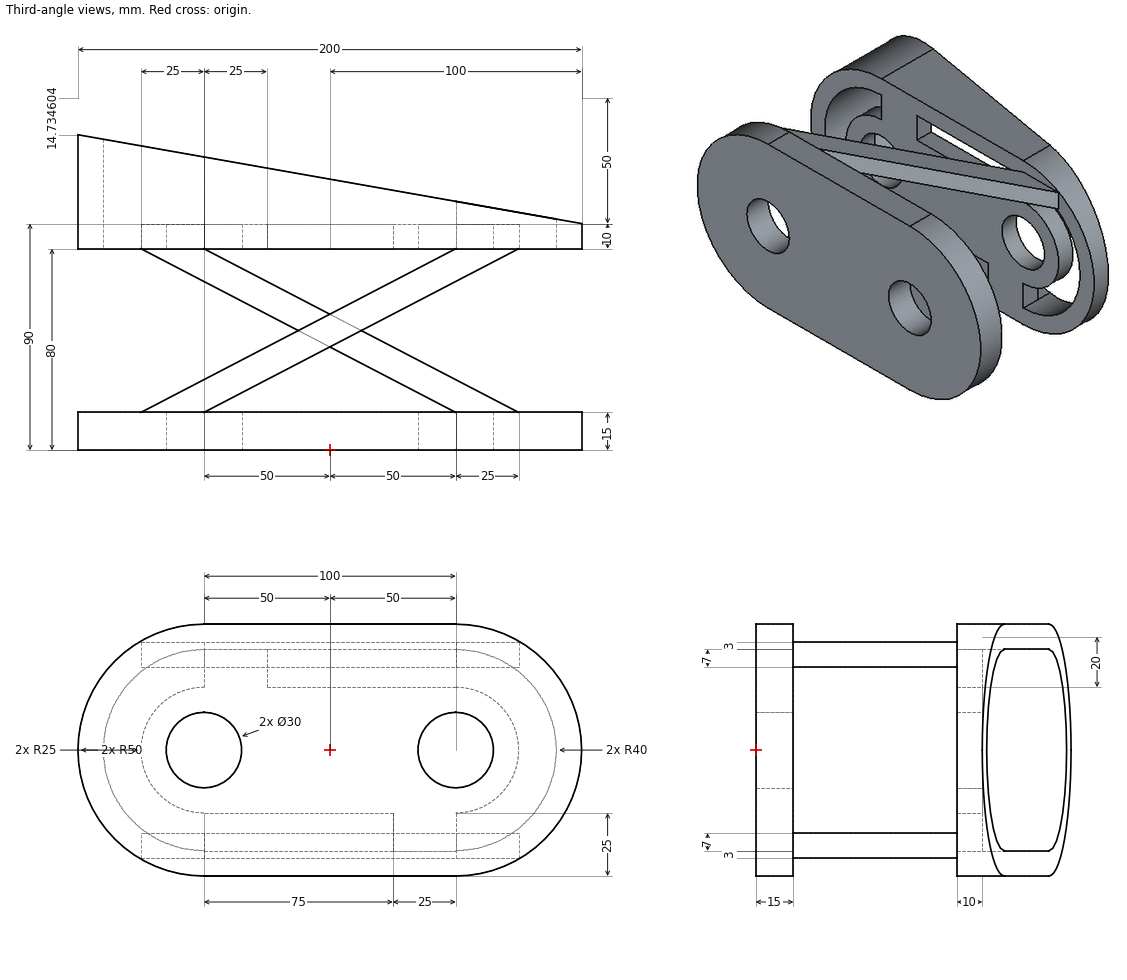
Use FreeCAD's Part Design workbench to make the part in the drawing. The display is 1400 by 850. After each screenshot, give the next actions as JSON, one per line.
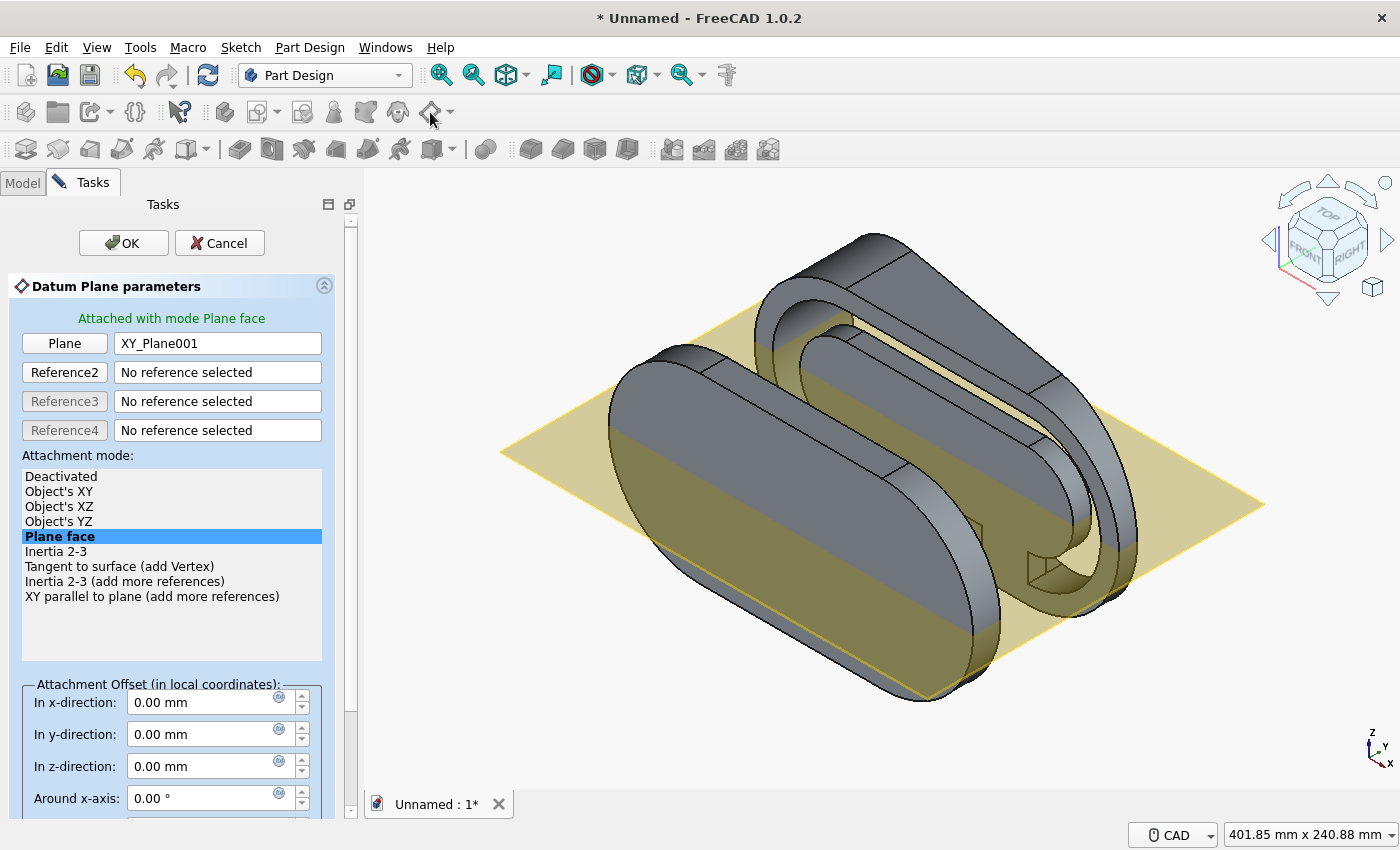
{"action": "triple_click", "coordinate": [210, 766]}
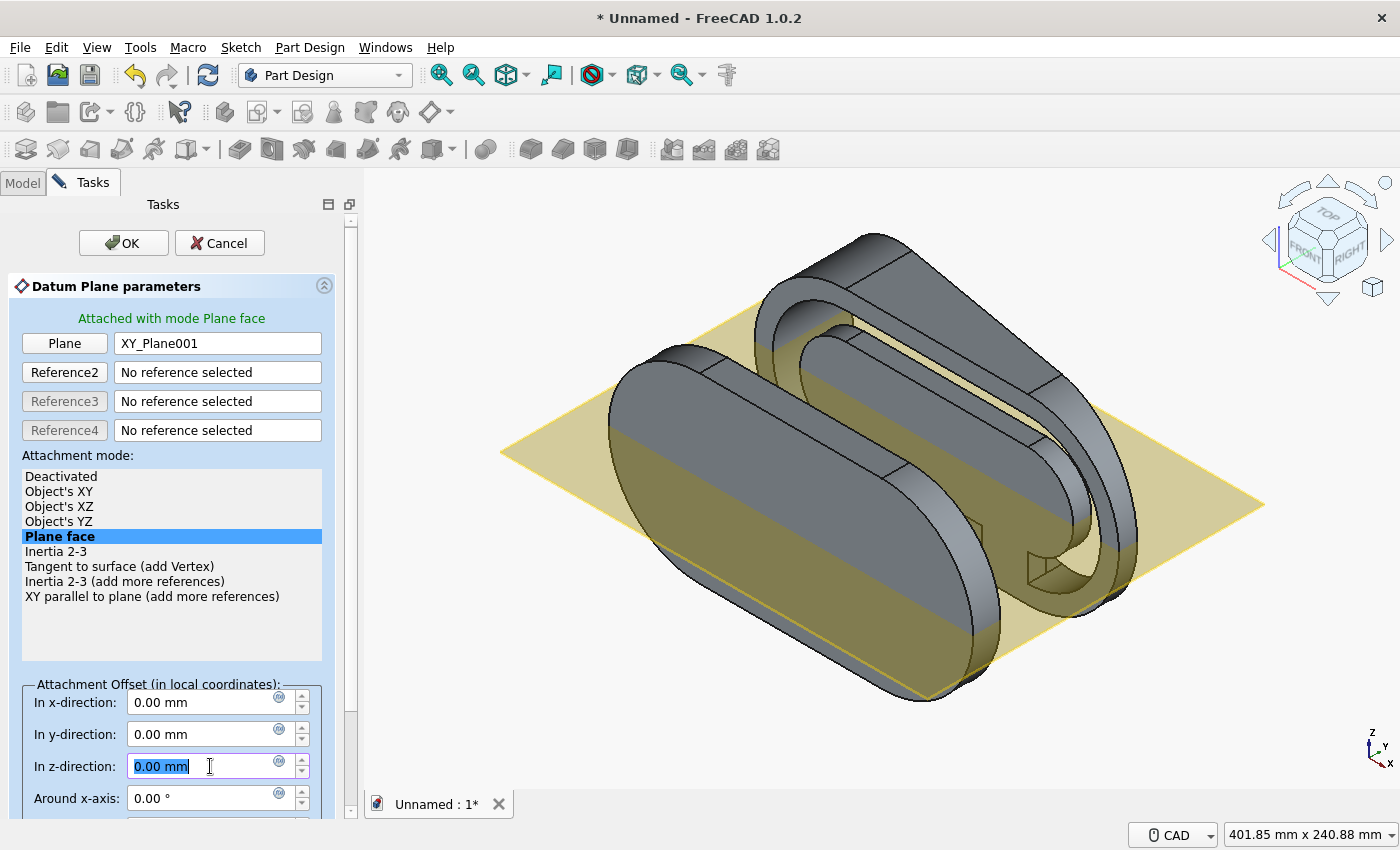
{"action": "type", "text": "25"}
{"action": "key", "text": "Tab"}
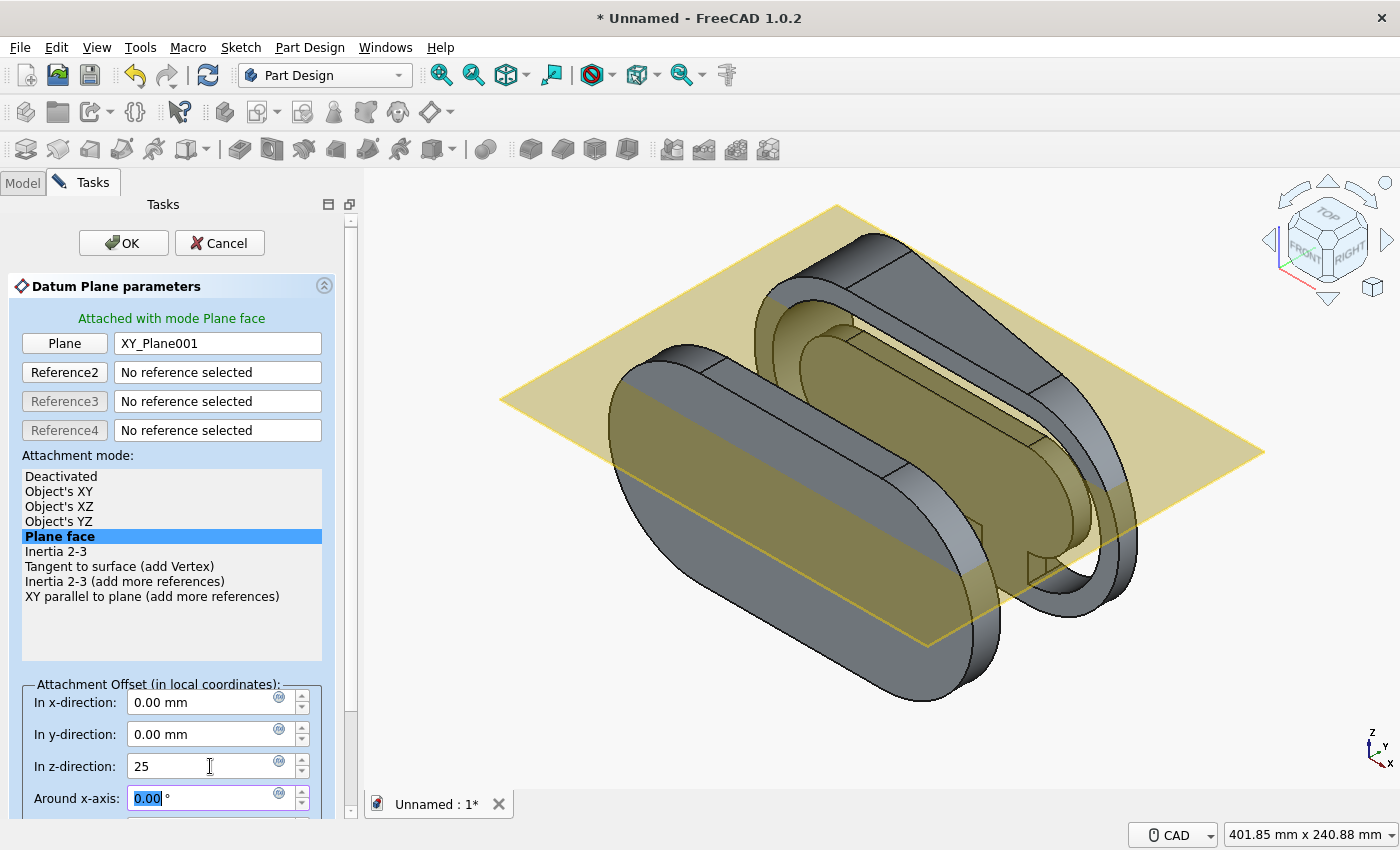
{"action": "left_click", "coordinate": [124, 243]}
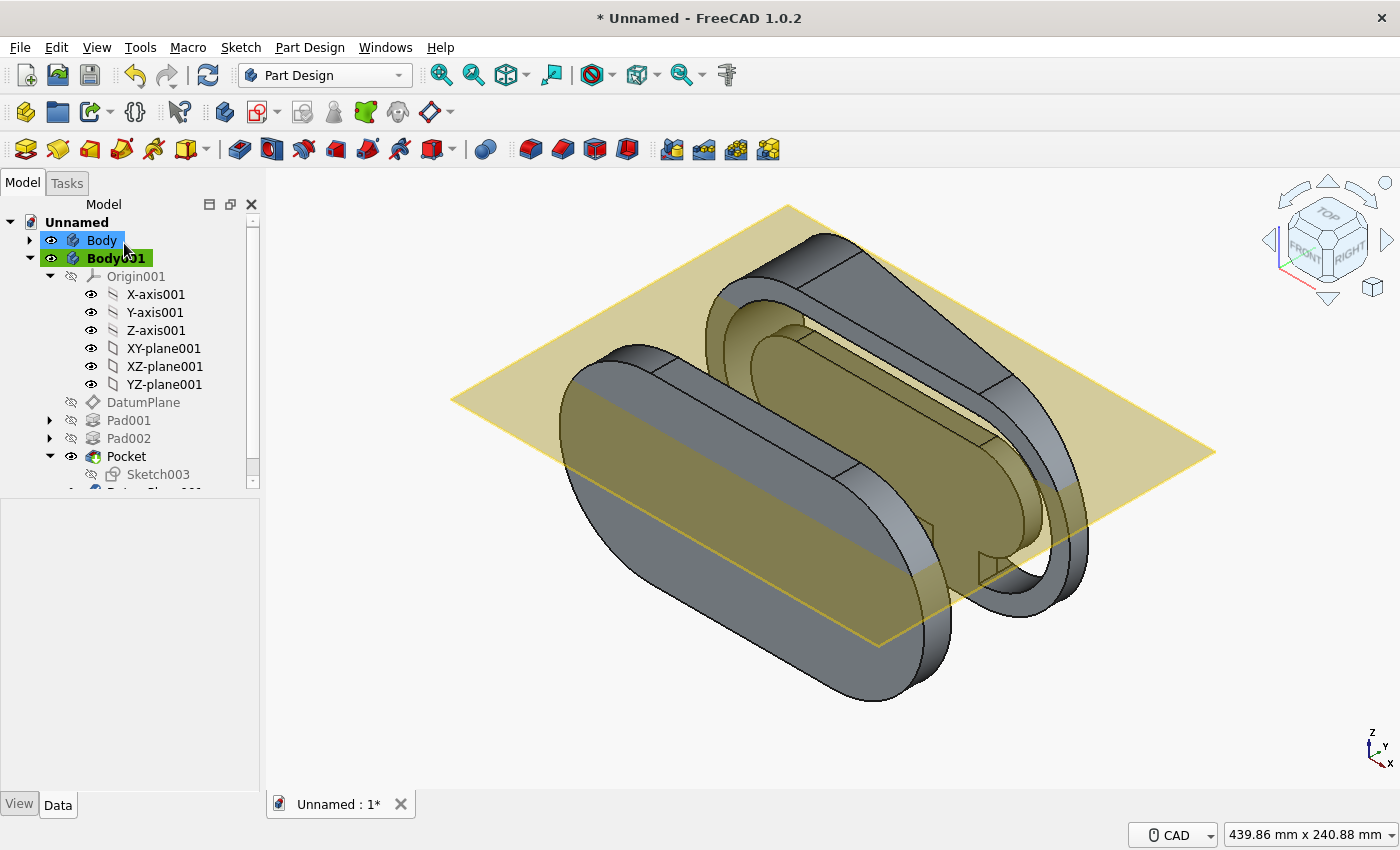
{"action": "scroll", "coordinate": [100, 344], "scroll_direction": "down", "scroll_amount": 3}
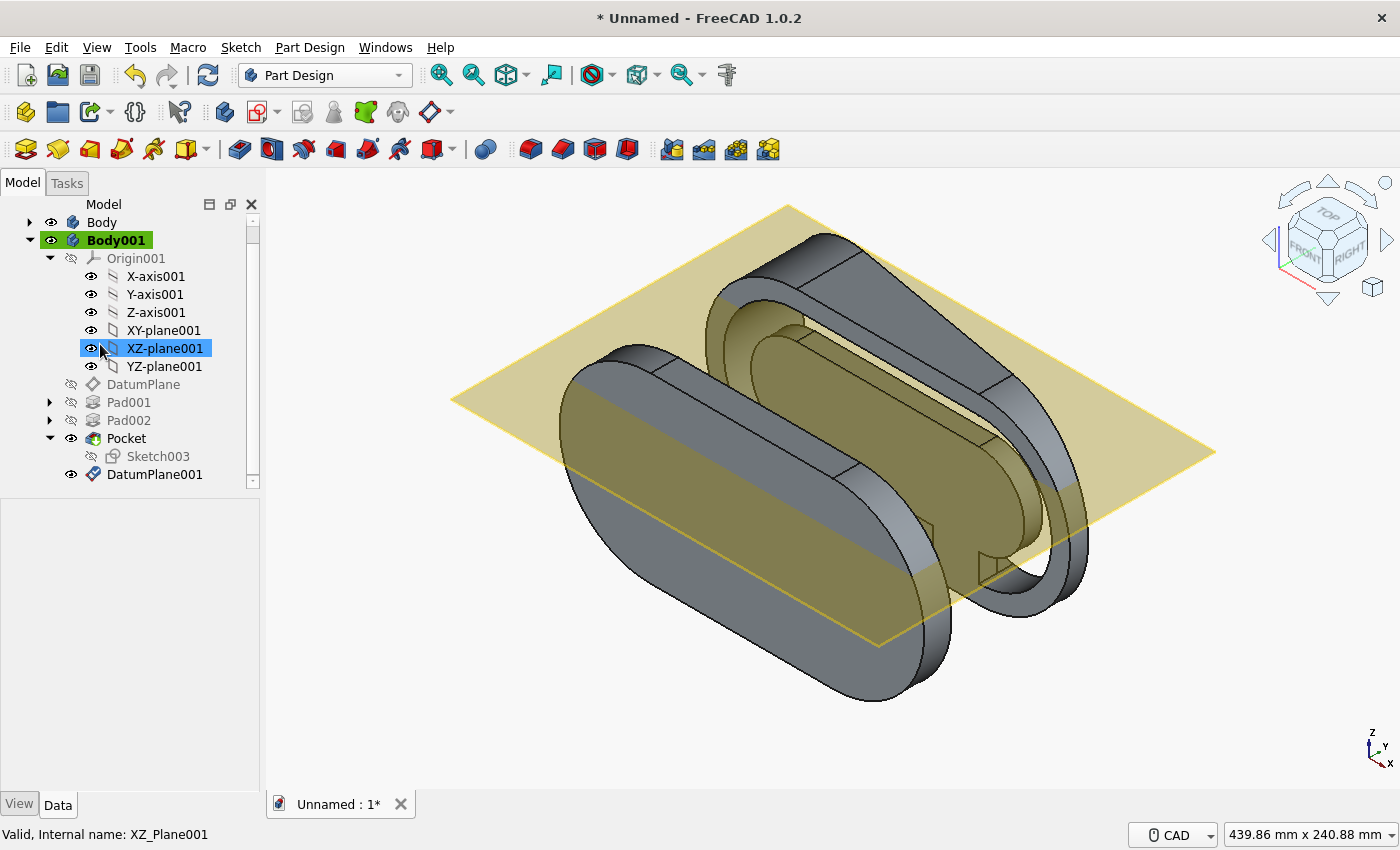
{"action": "left_click", "coordinate": [116, 474]}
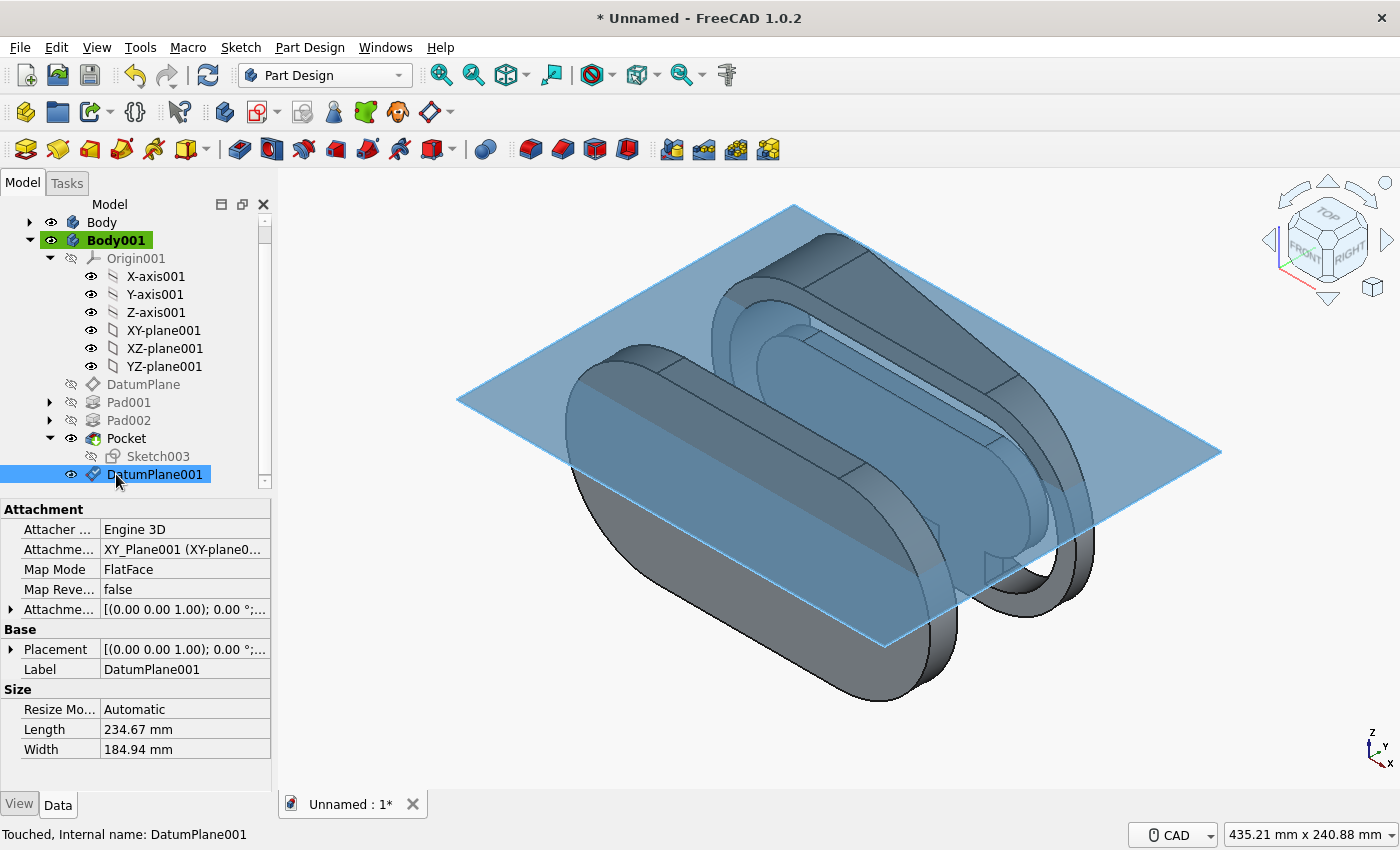
{"action": "left_click", "coordinate": [258, 112]}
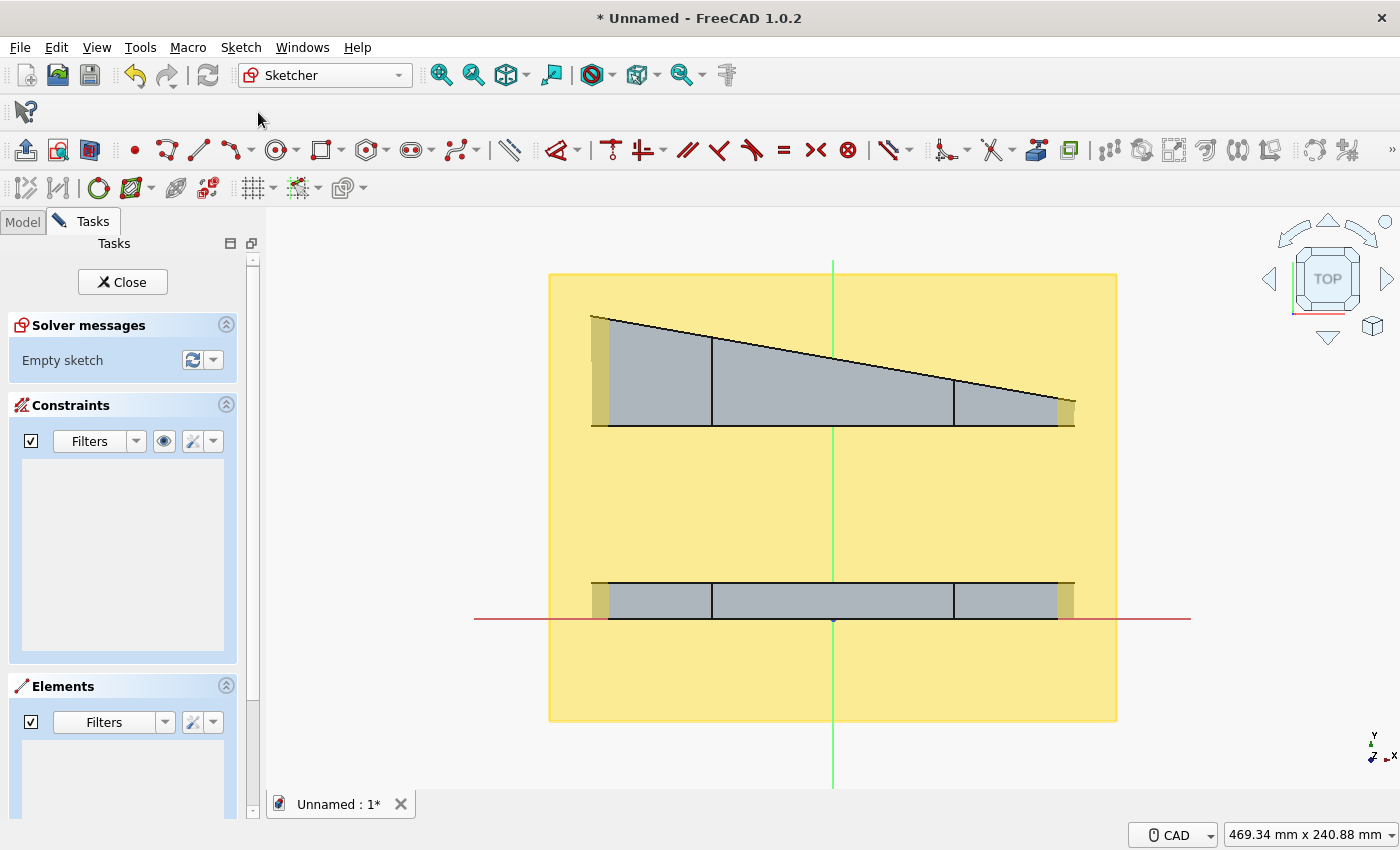
{"action": "left_click", "coordinate": [90, 150]}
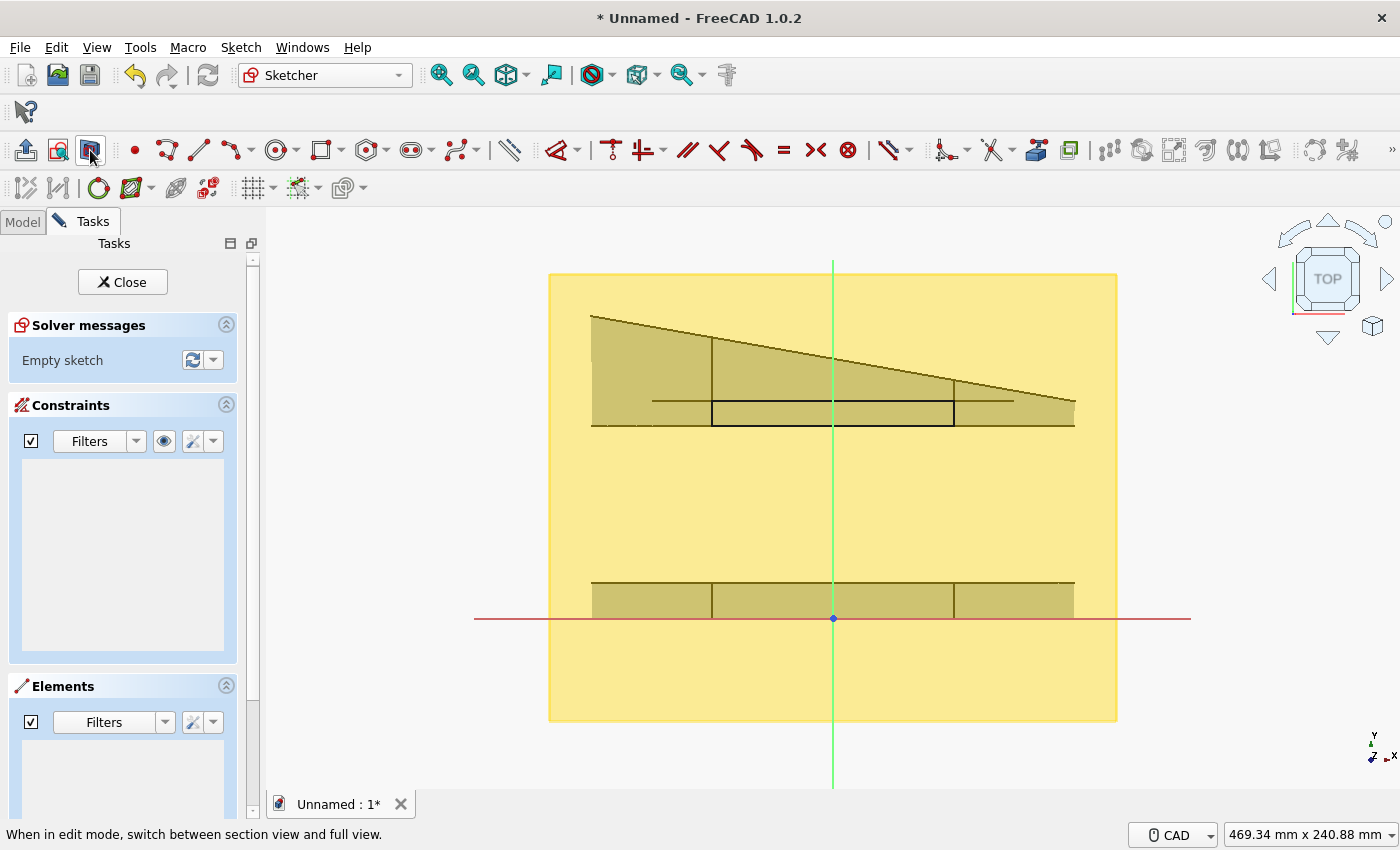
{"action": "scroll", "coordinate": [740, 405], "scroll_direction": "up", "scroll_amount": 12}